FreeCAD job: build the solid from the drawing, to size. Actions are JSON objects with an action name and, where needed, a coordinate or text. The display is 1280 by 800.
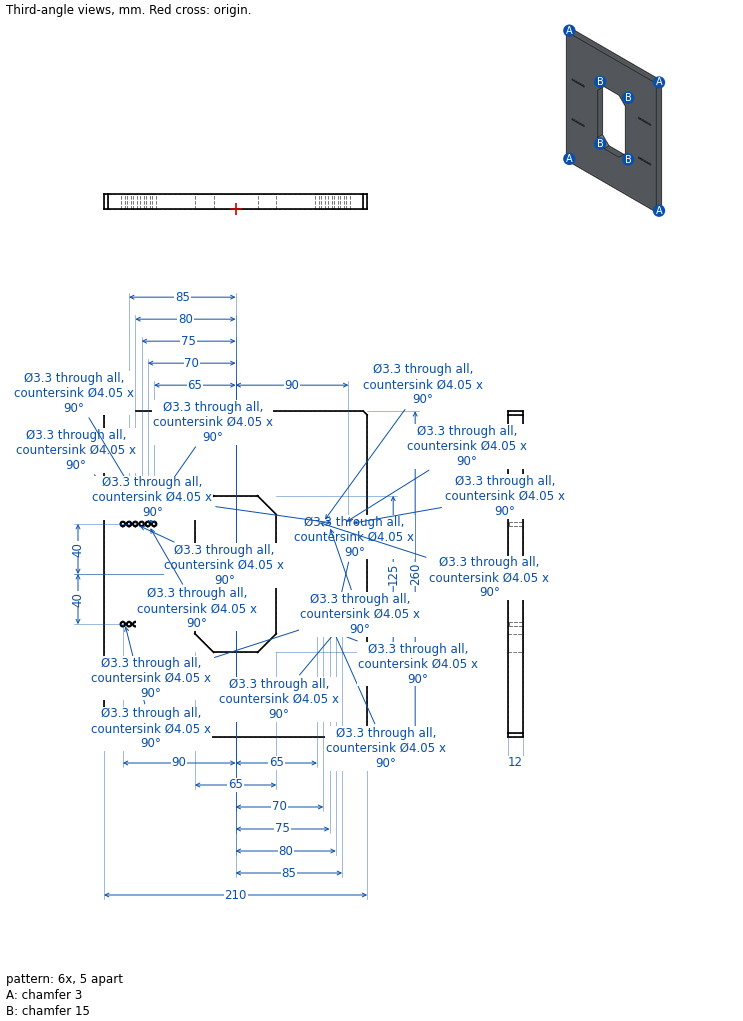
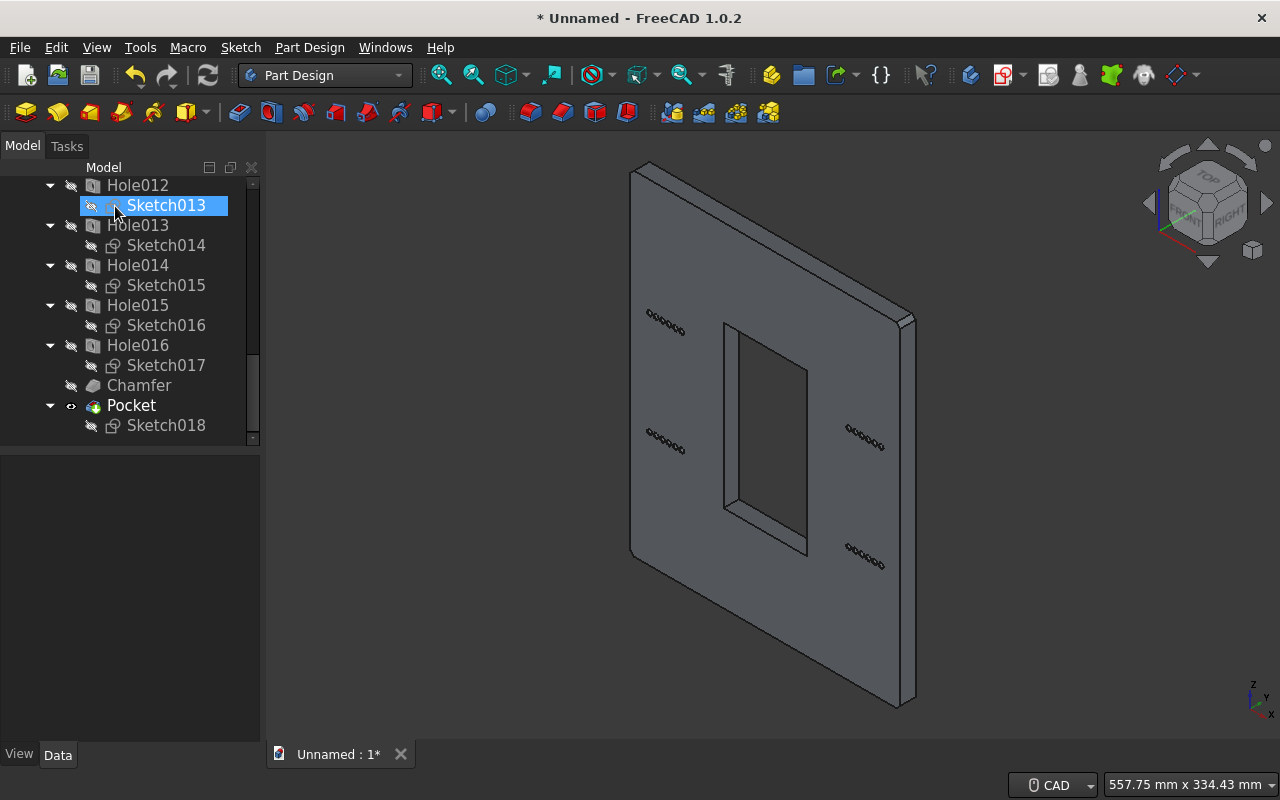
{"action": "scroll", "coordinate": [731, 503], "scroll_direction": "up", "scroll_amount": 4}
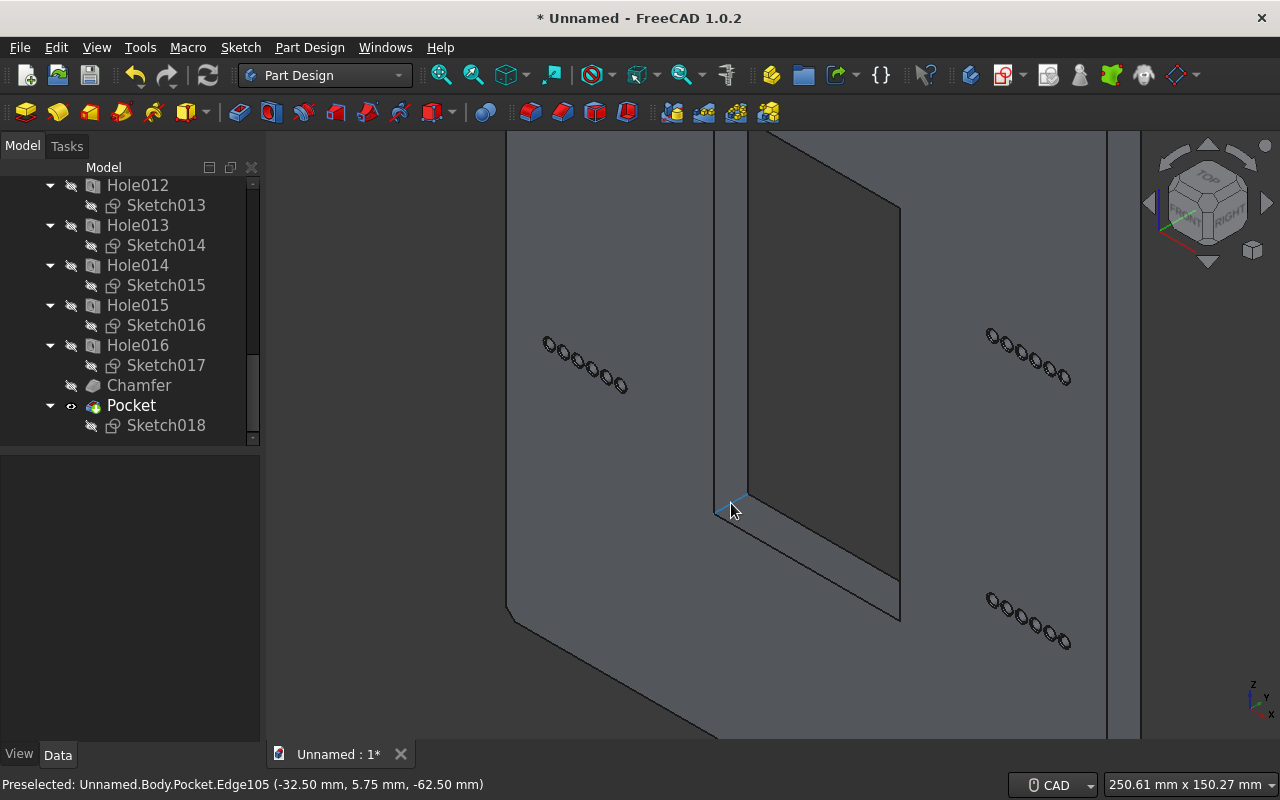
{"action": "left_click", "coordinate": [442, 76]}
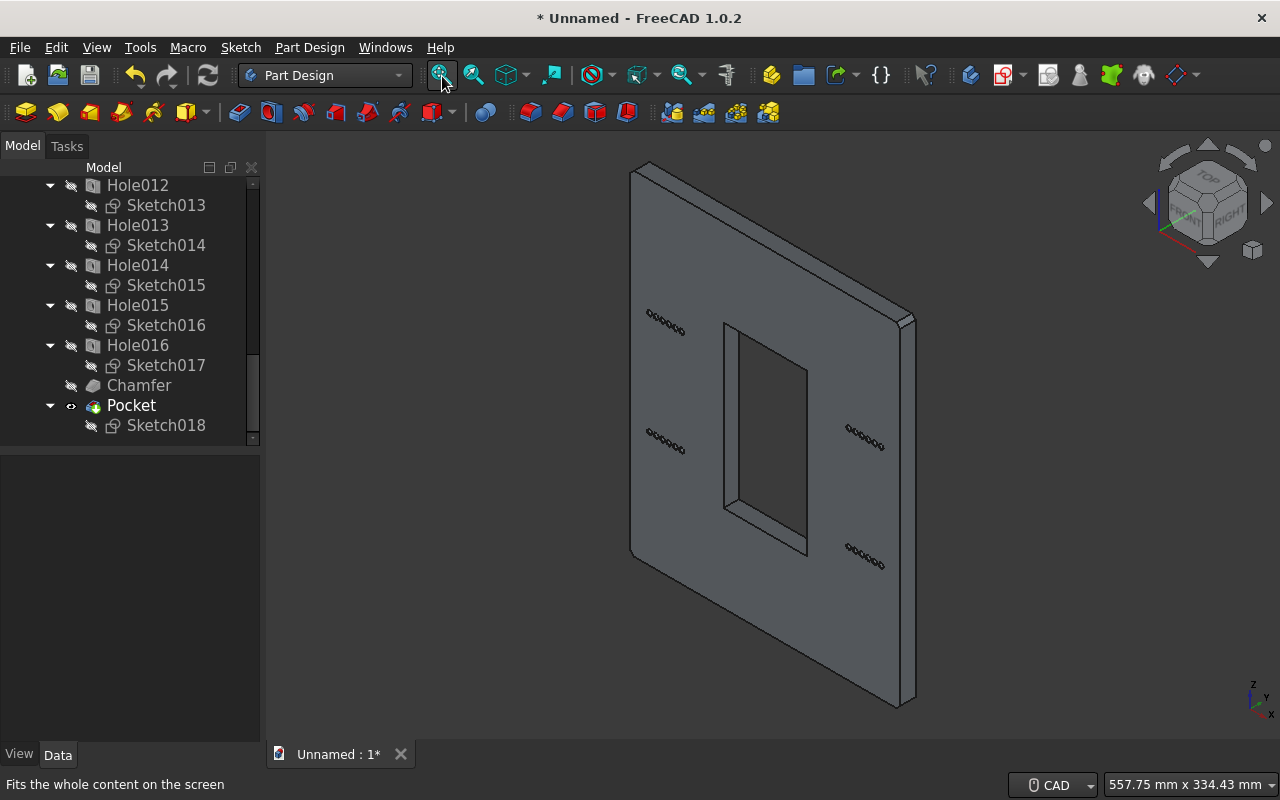
{"action": "key", "text": "2"}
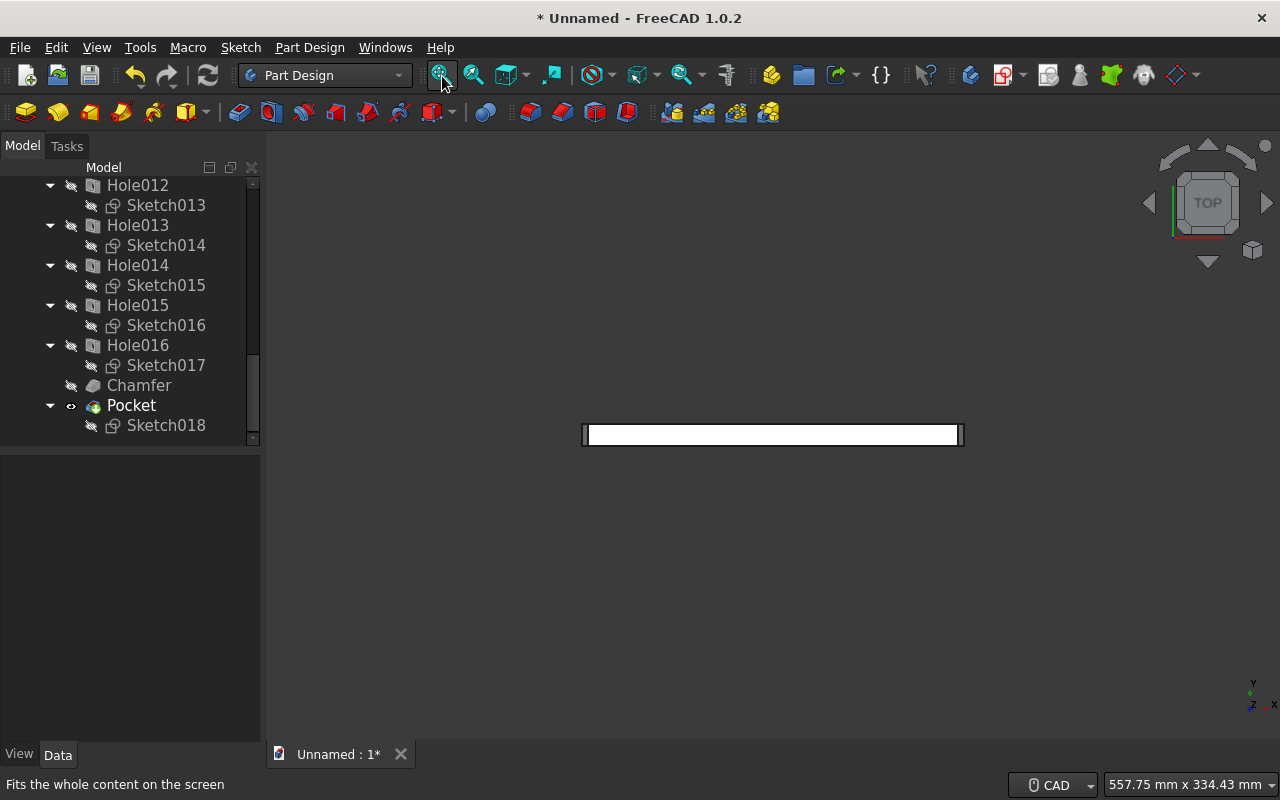
{"action": "left_click", "coordinate": [442, 76]}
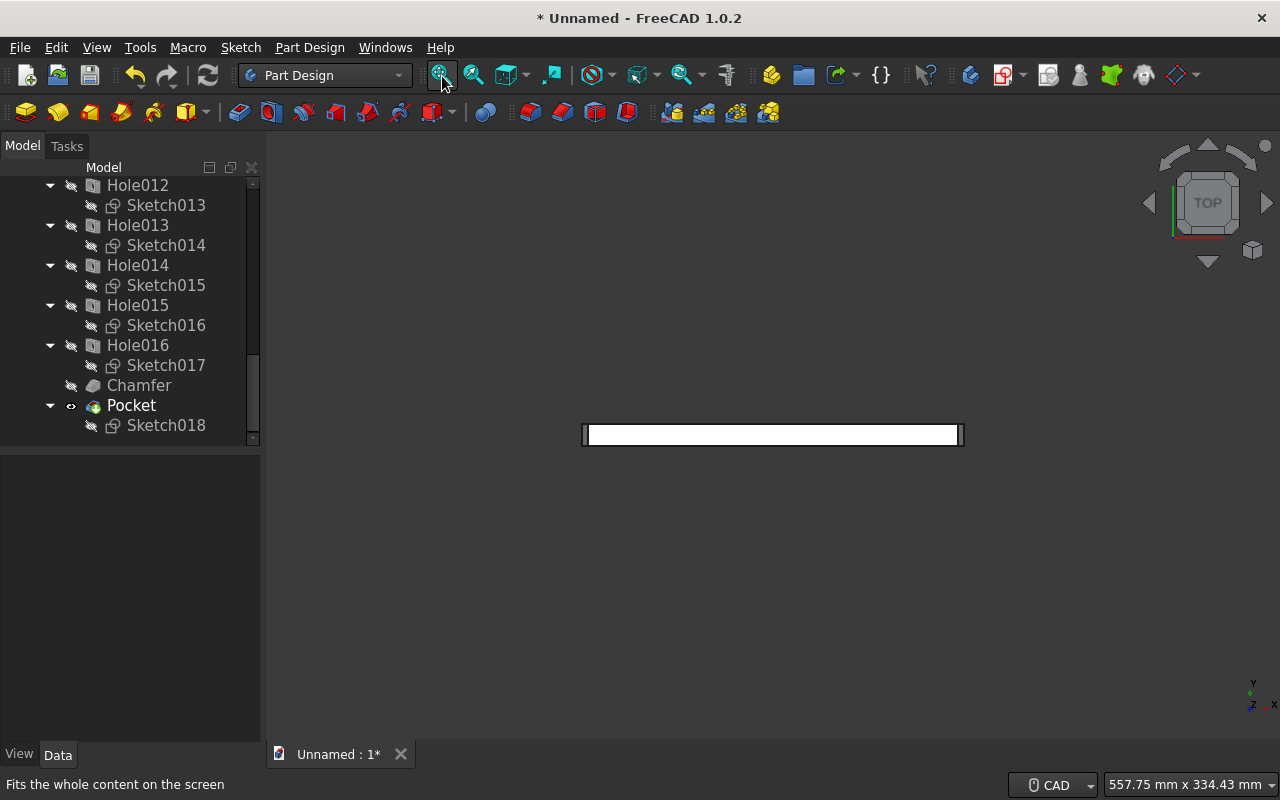
{"action": "scroll", "coordinate": [714, 434], "scroll_direction": "up", "scroll_amount": 4}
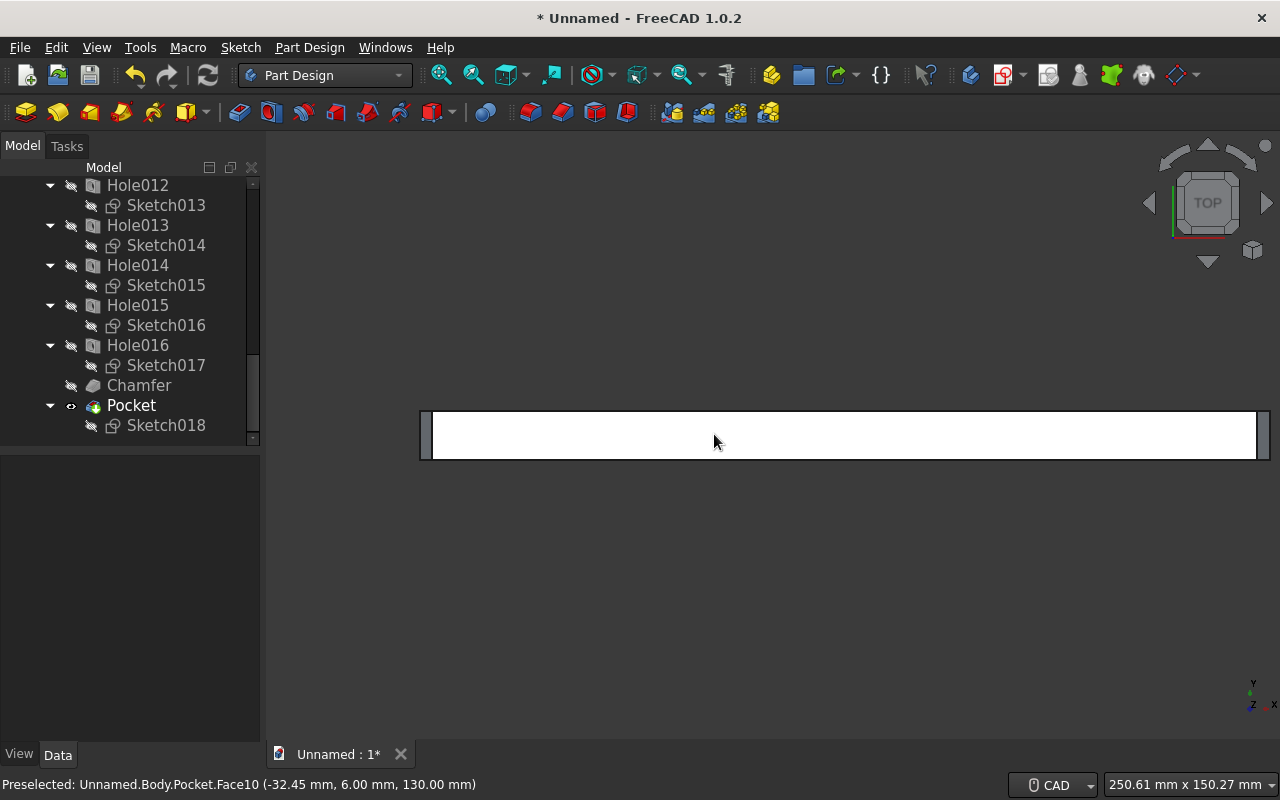
{"action": "left_click", "coordinate": [442, 76]}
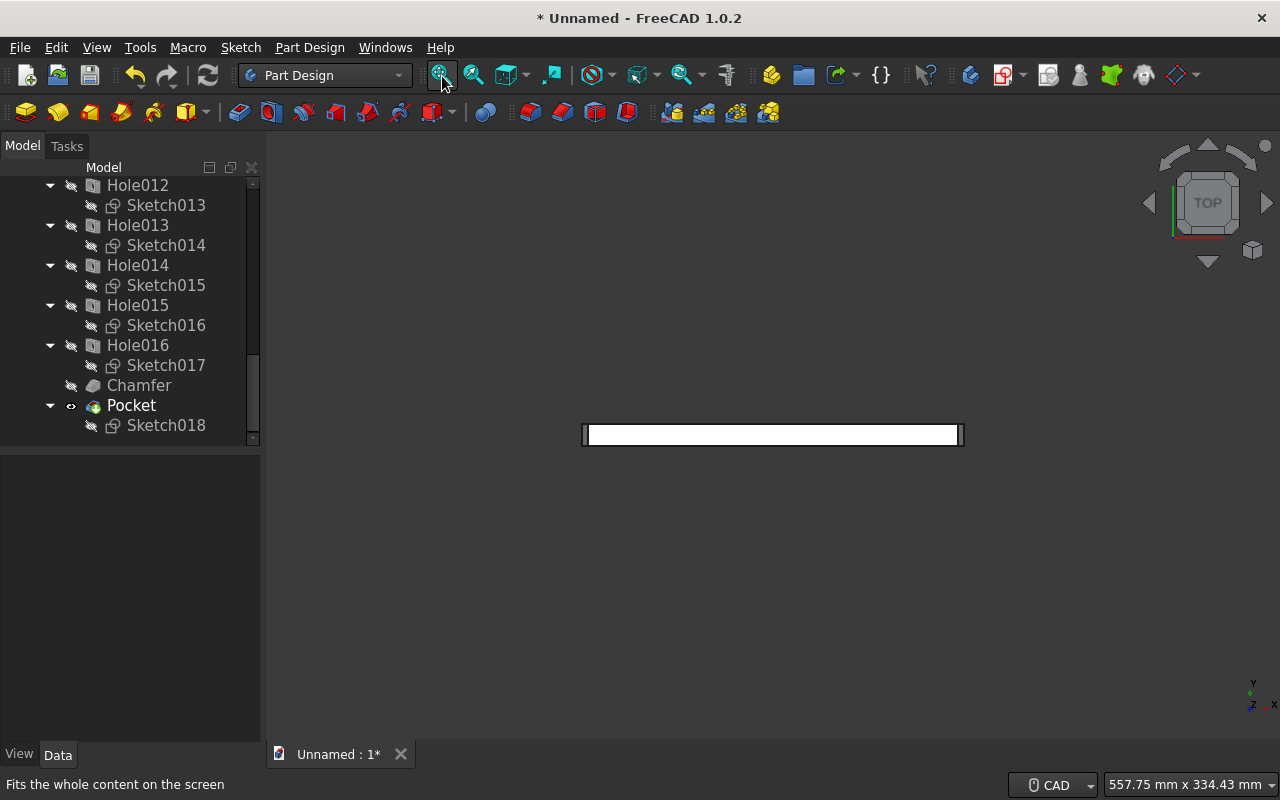
{"action": "key", "text": "0"}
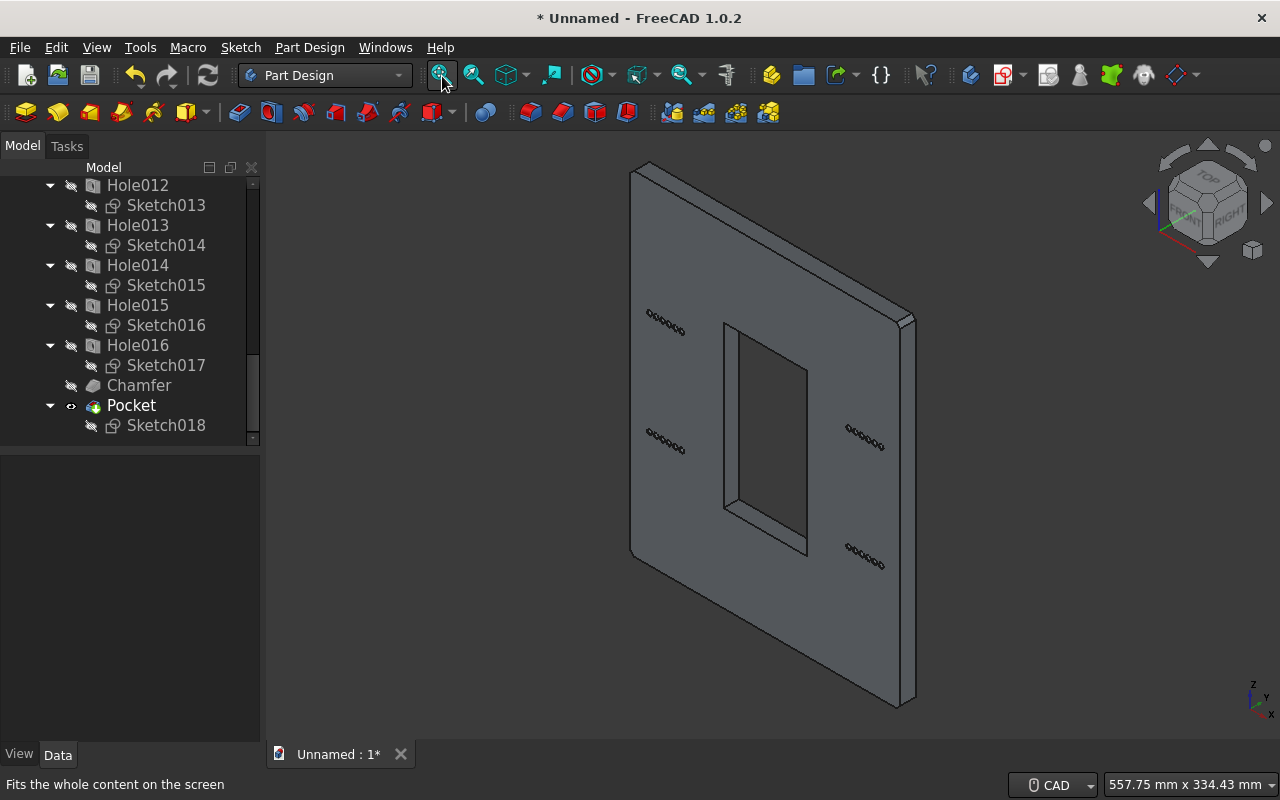
{"action": "scroll", "coordinate": [731, 503], "scroll_direction": "up", "scroll_amount": 4}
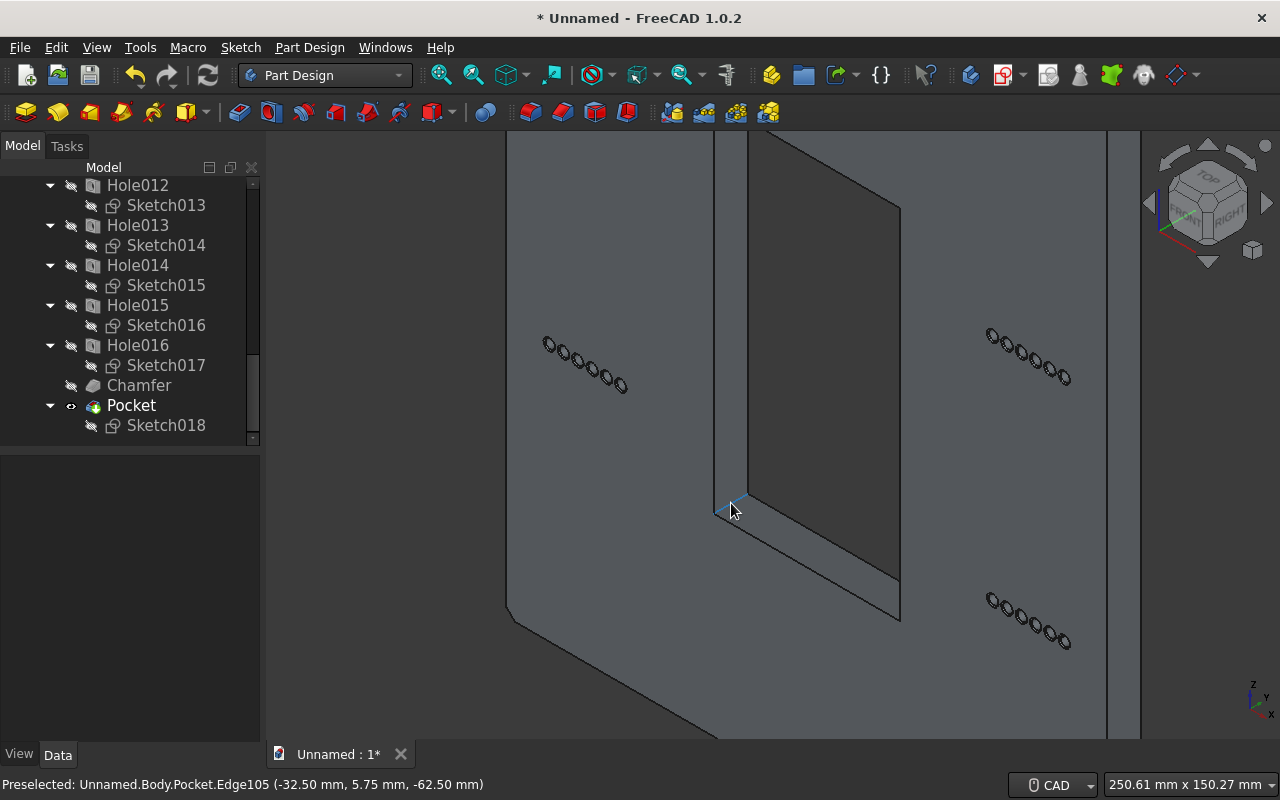
{"action": "left_click", "coordinate": [442, 76]}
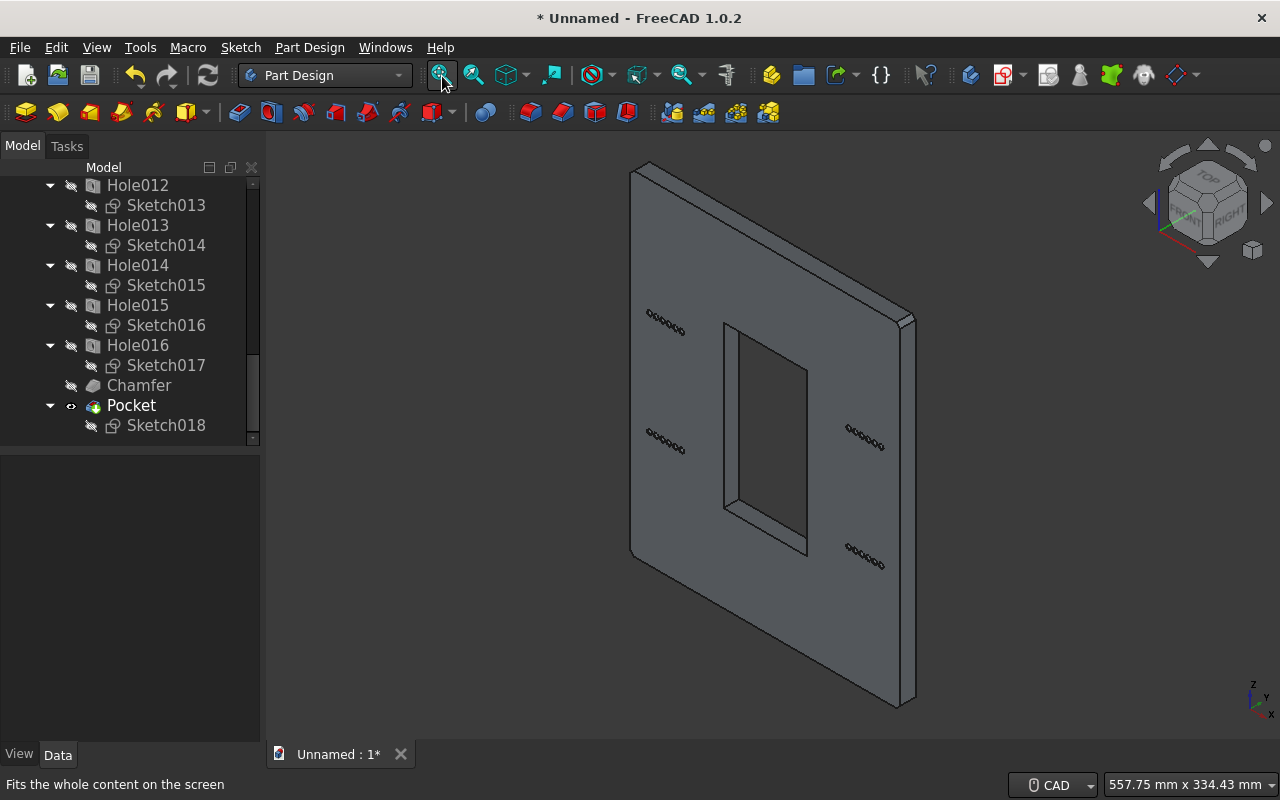
{"action": "key", "text": "1"}